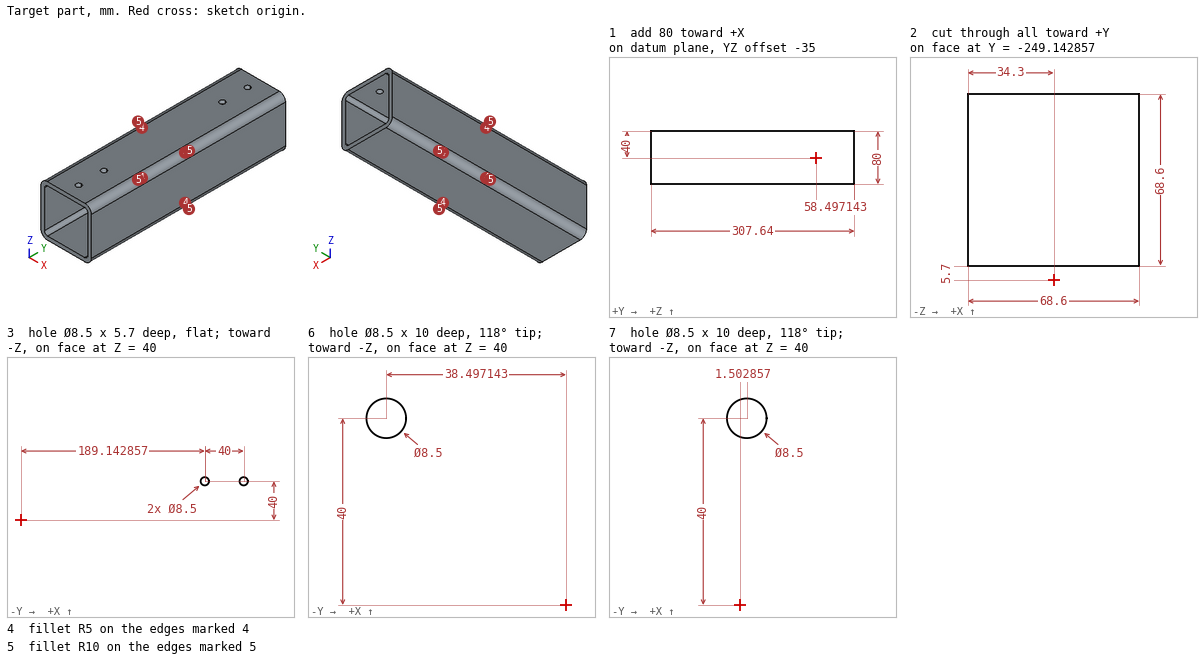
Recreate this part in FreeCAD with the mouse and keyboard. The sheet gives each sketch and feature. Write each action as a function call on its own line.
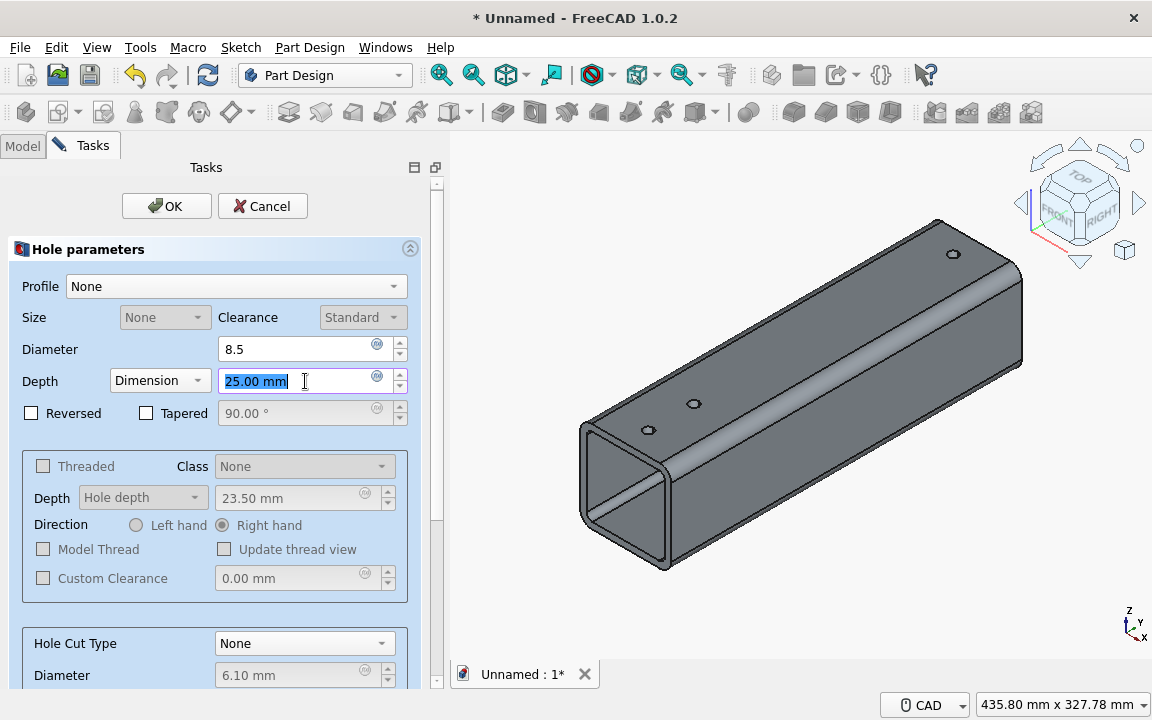
text(10)
key(Tab)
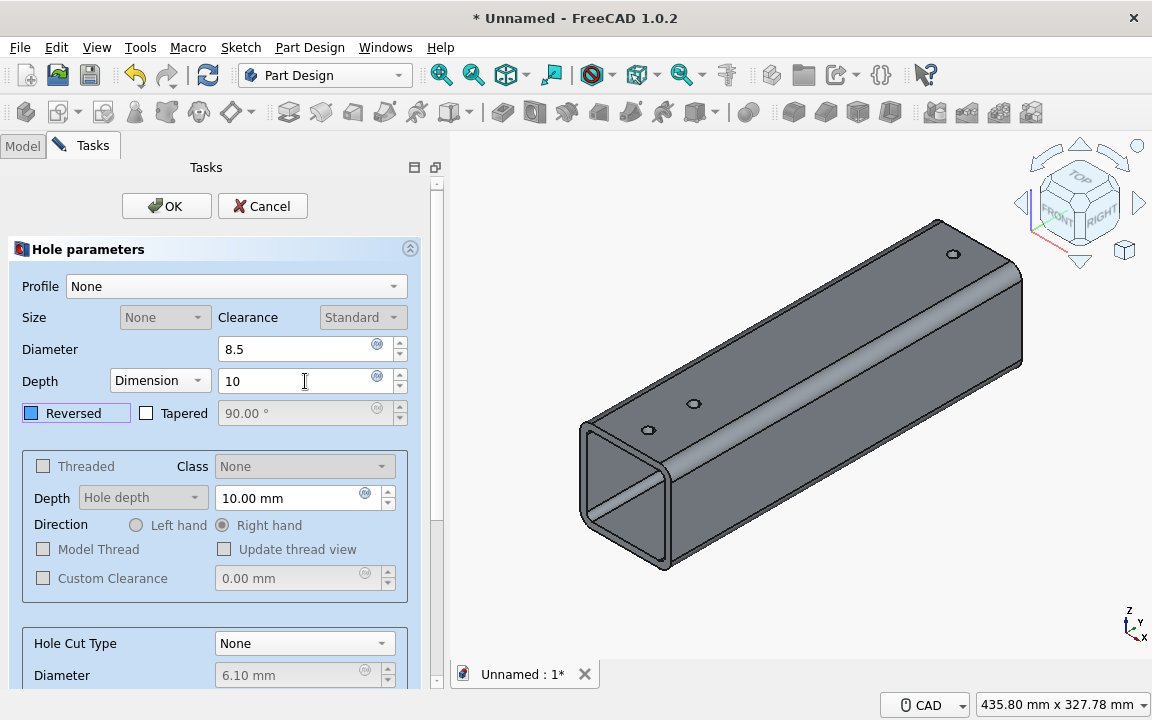
click(167, 206)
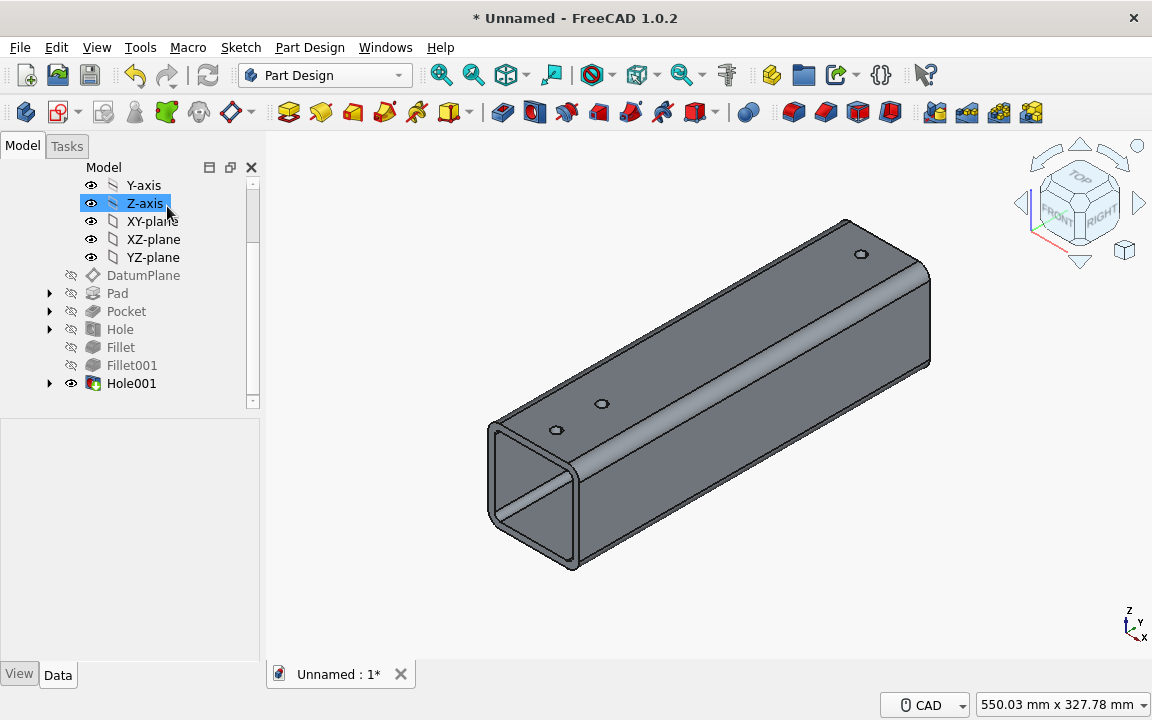
click(709, 341)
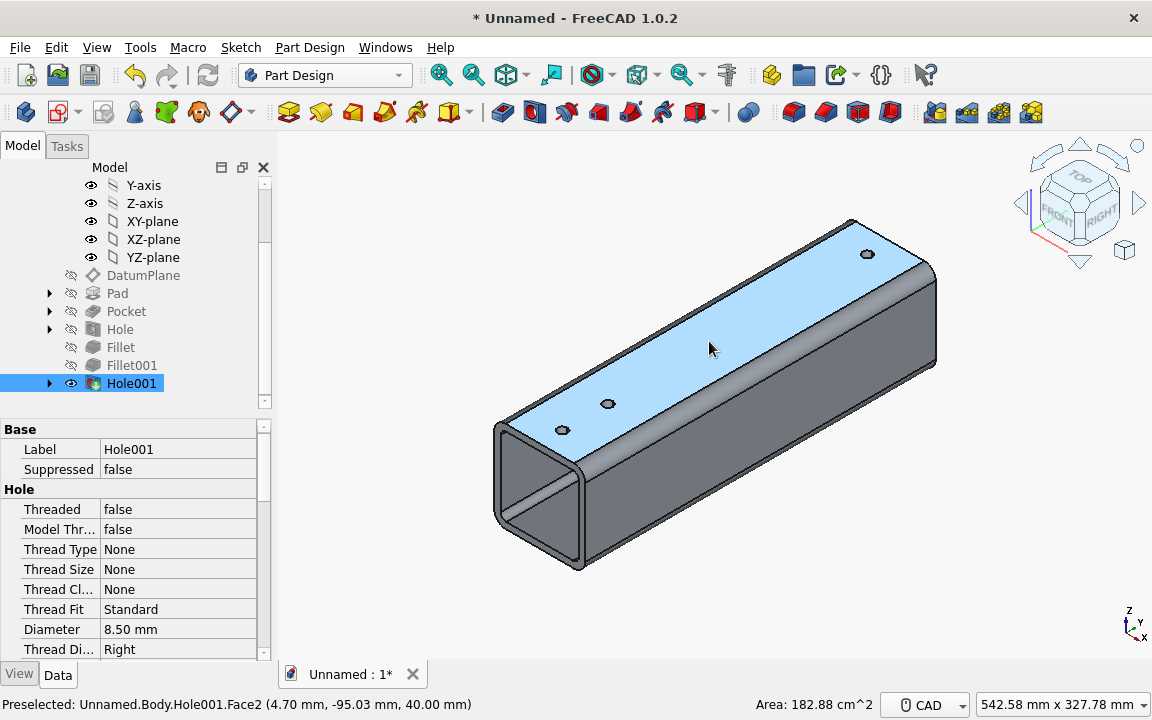
click(58, 112)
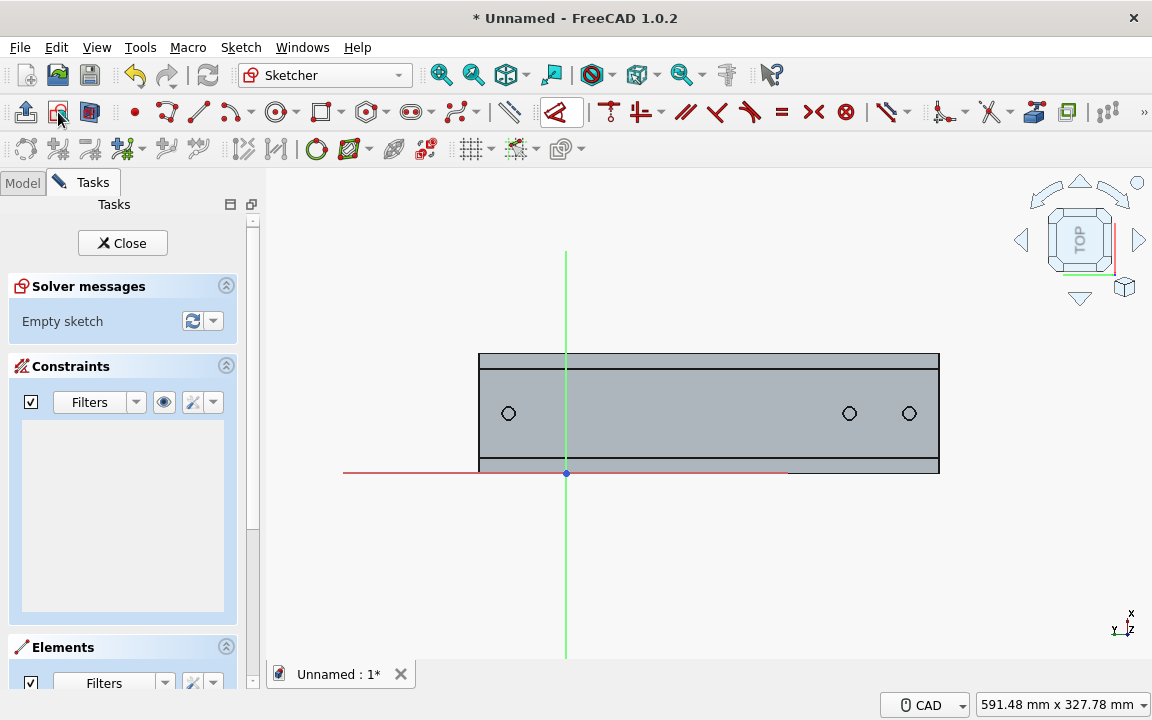
scroll(565, 414, up, 15)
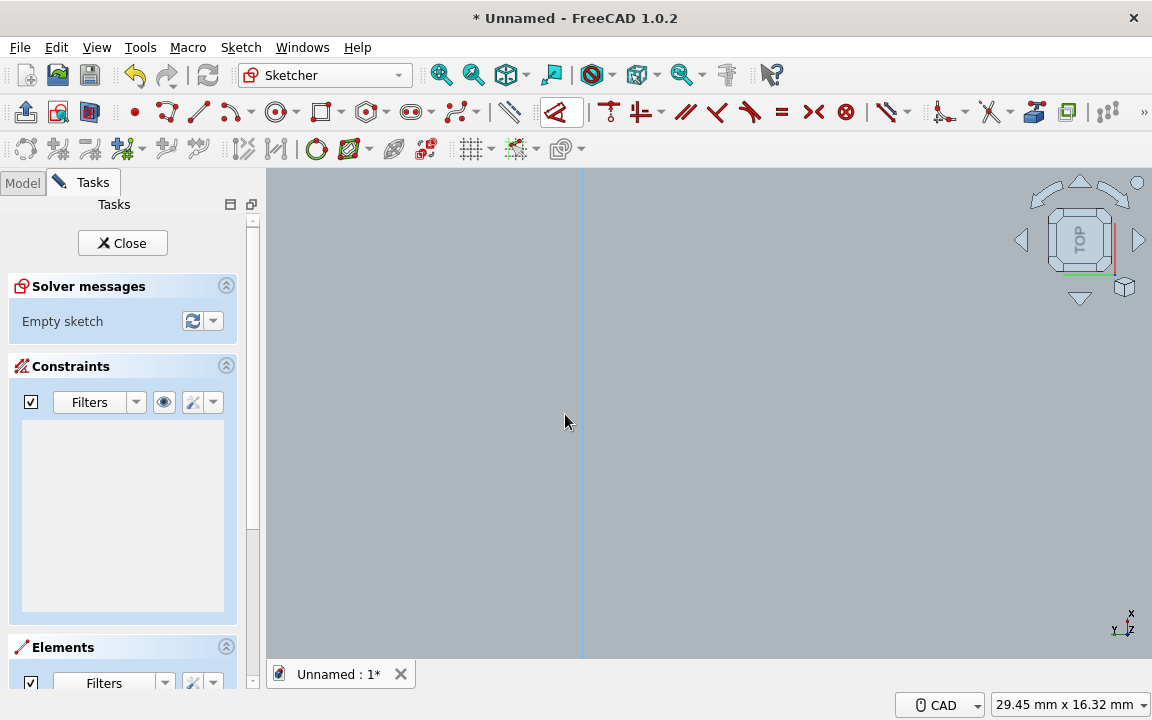
click(276, 112)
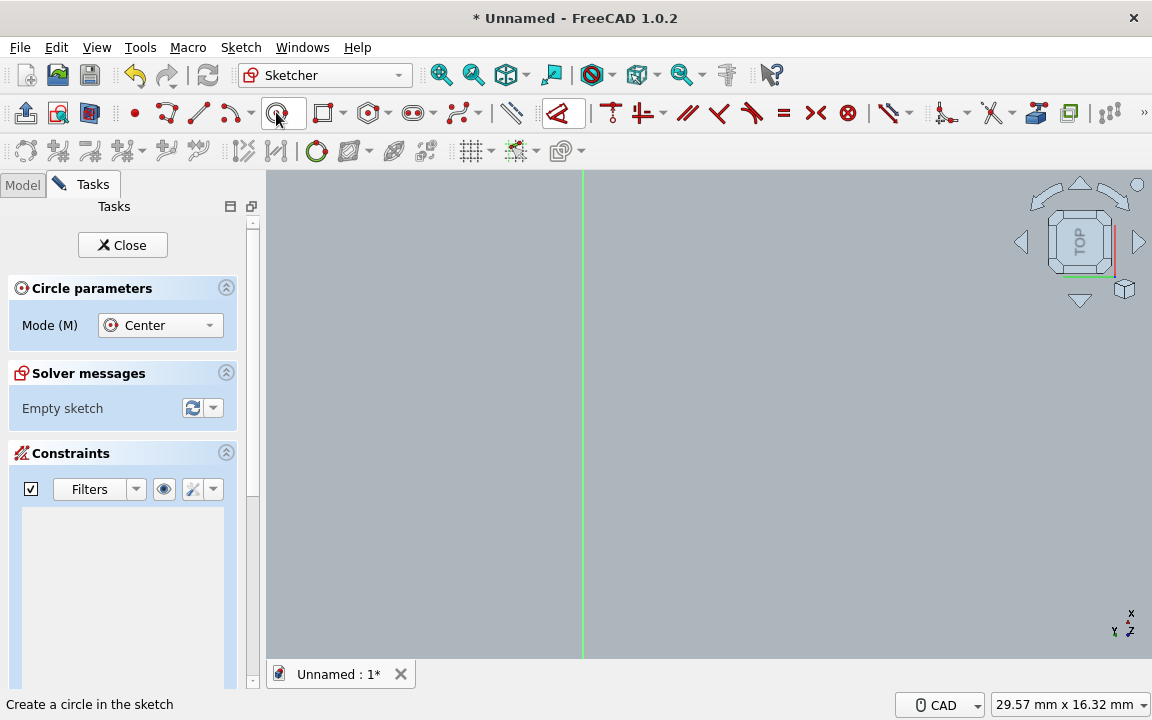
click(628, 395)
move(718, 305)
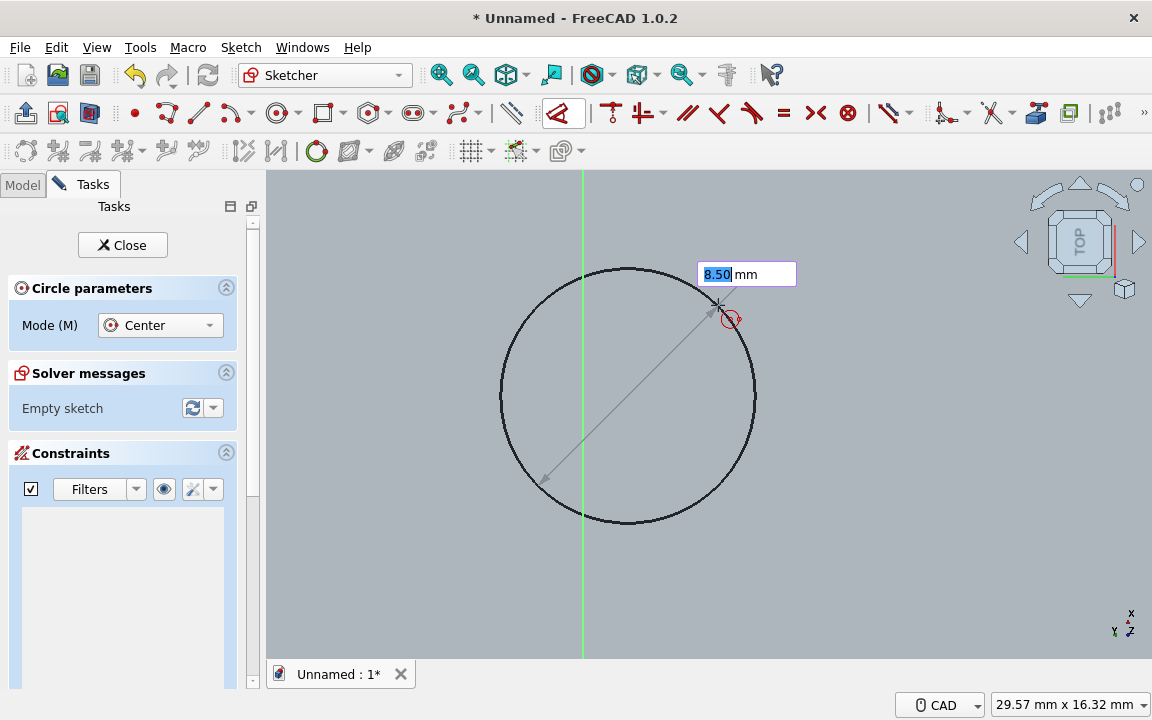
text(8.5)
key(Return)
key(Escape)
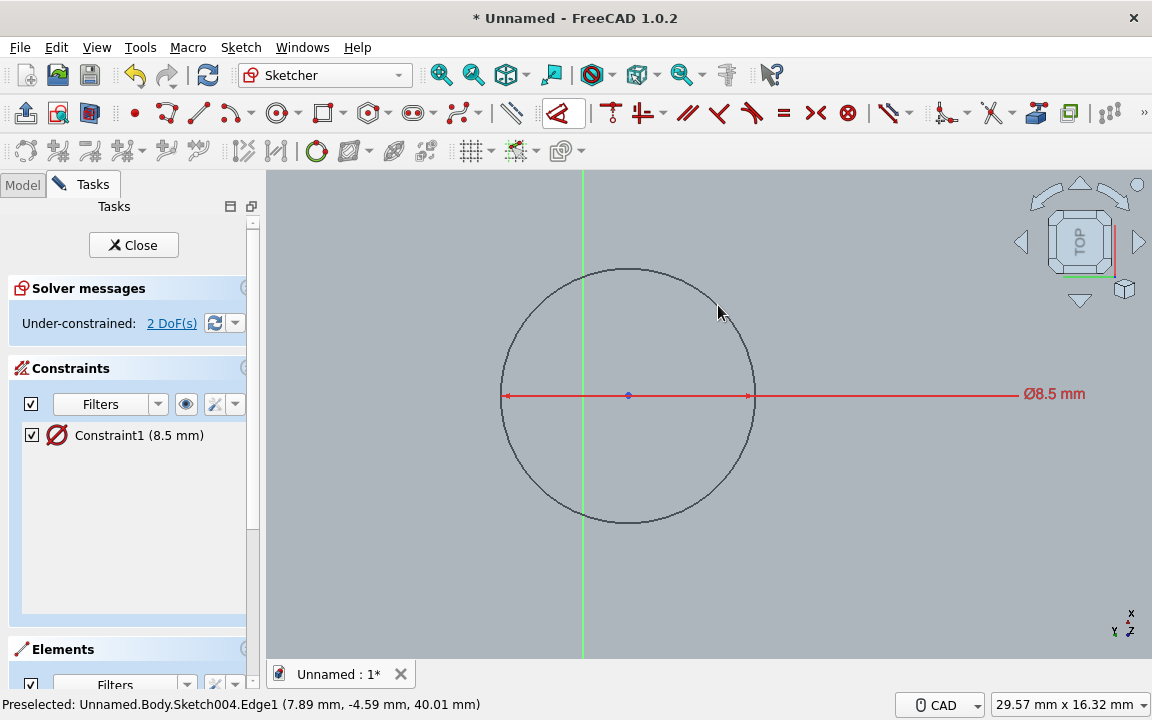
click(628, 396)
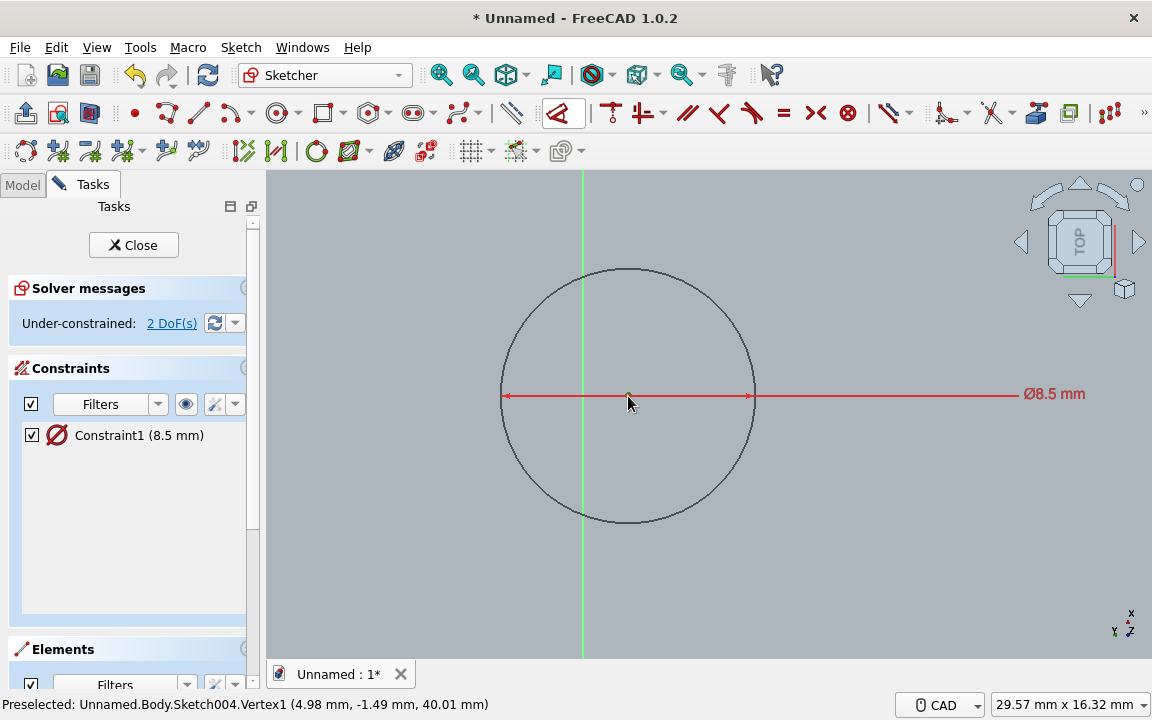
key(i)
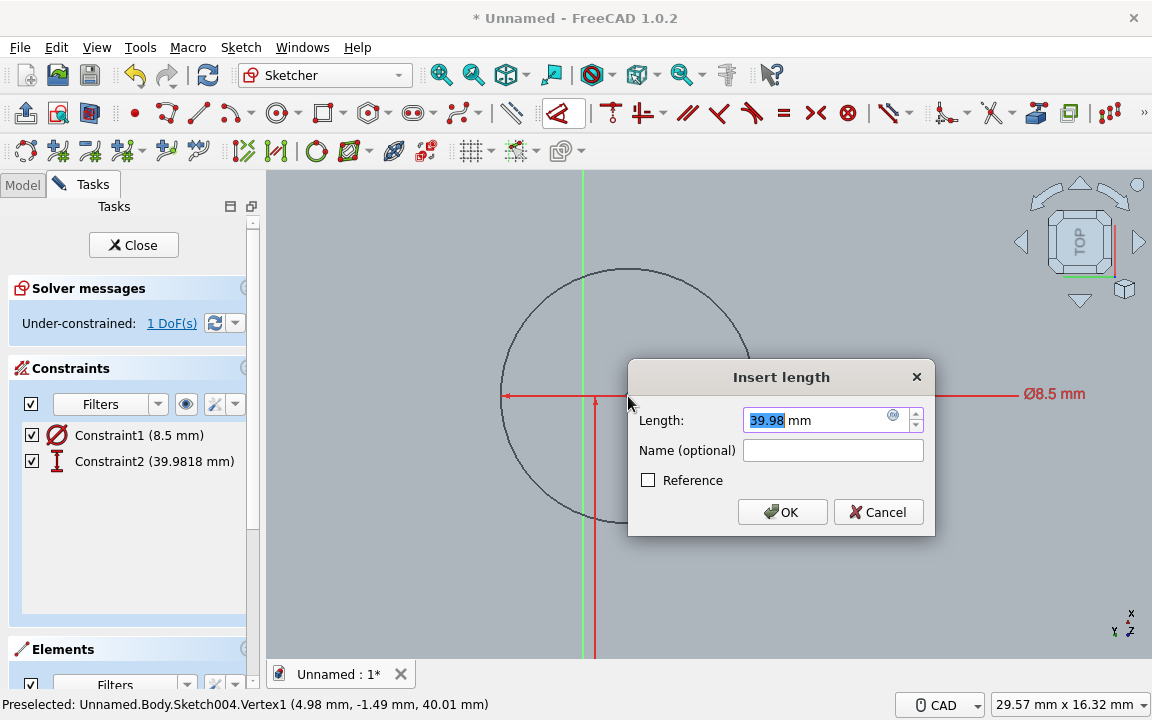
text(40)
key(Return)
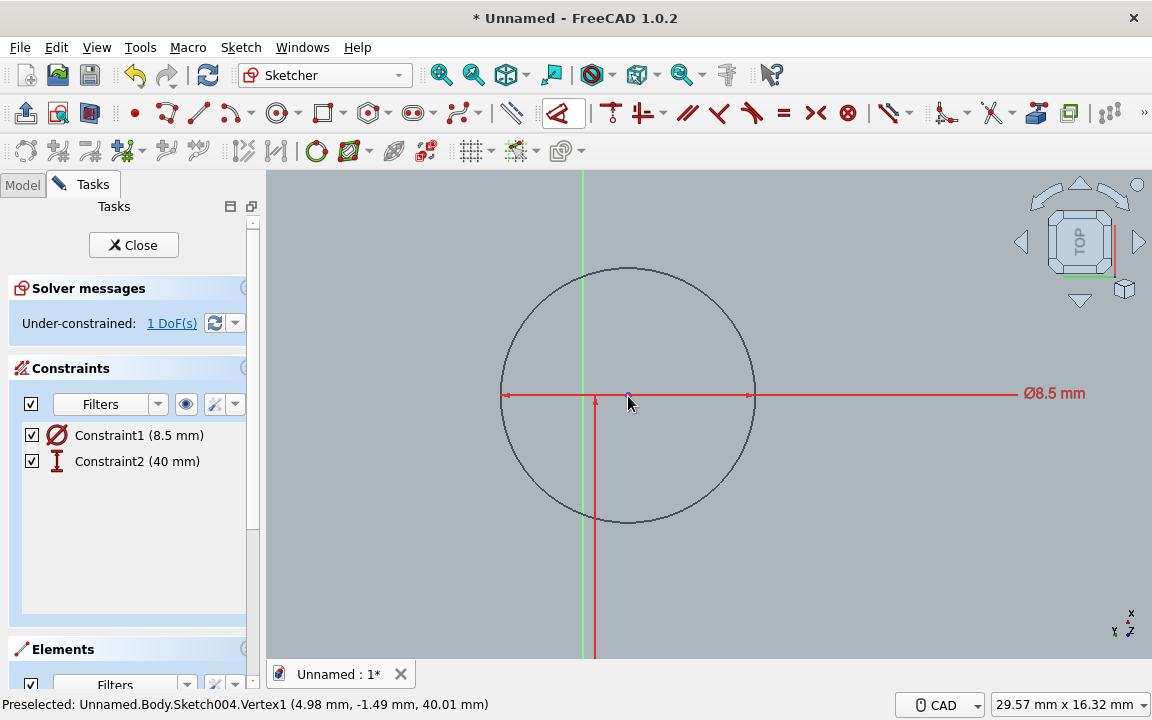
click(628, 395)